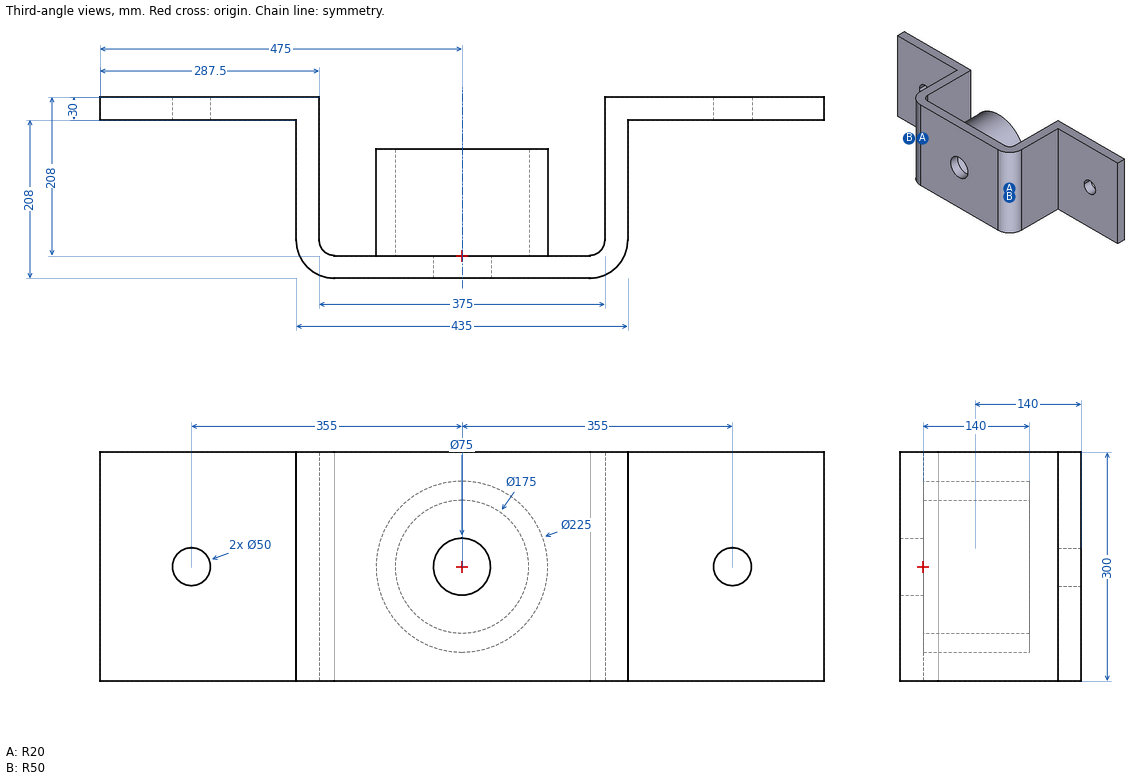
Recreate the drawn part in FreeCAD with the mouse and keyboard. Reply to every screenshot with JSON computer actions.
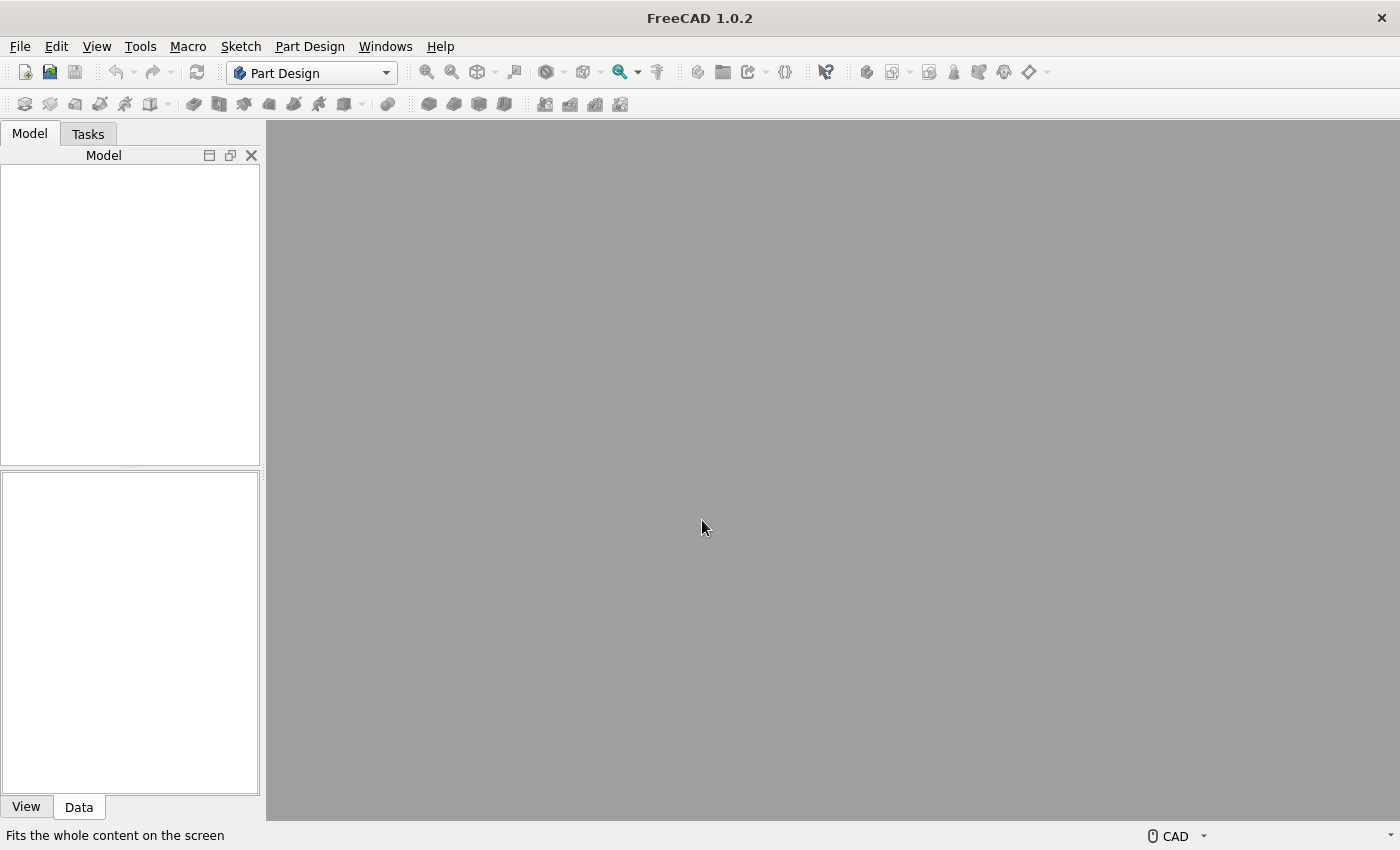
{"action": "left_click", "coordinate": [25, 72]}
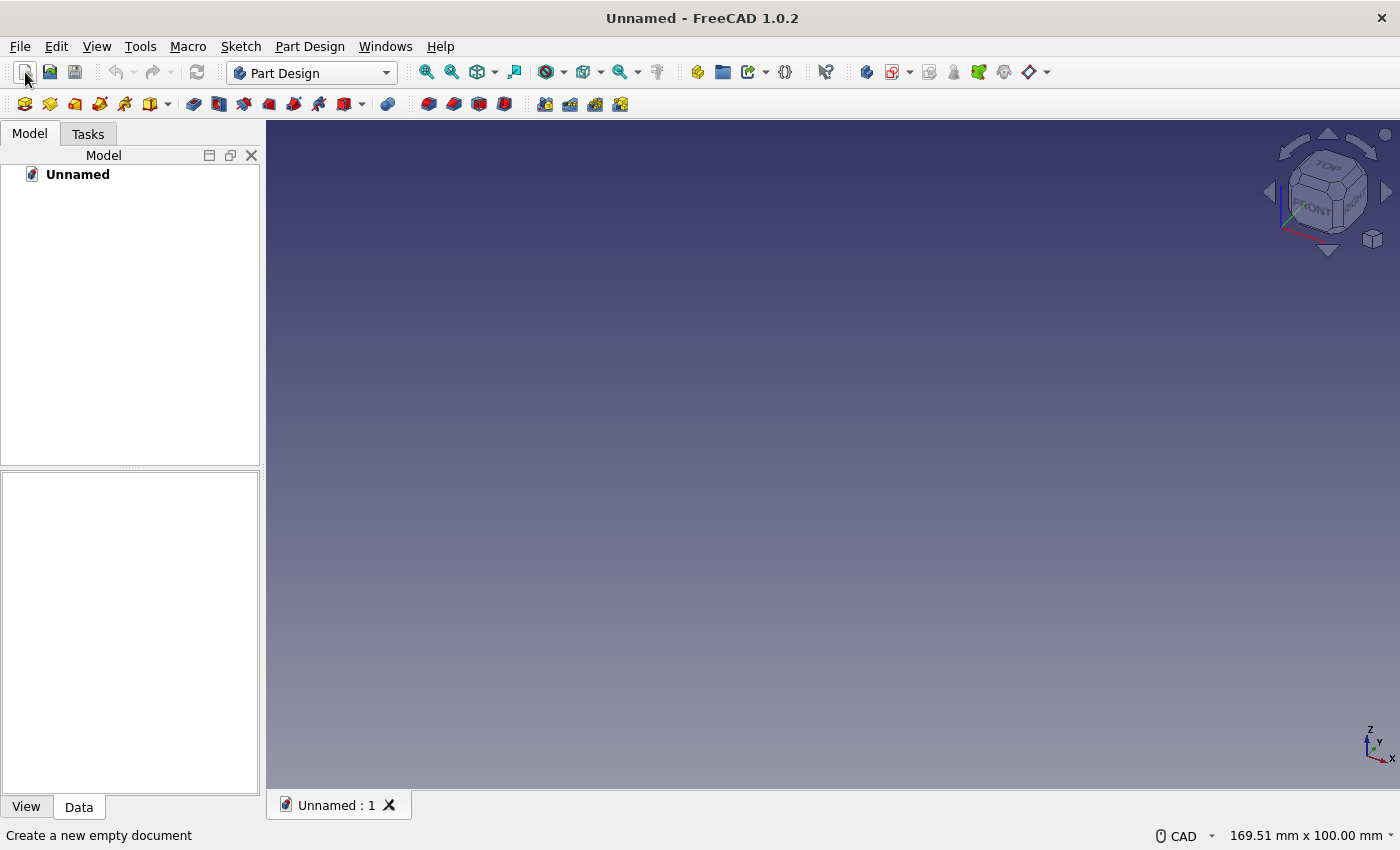
{"action": "left_click", "coordinate": [892, 72]}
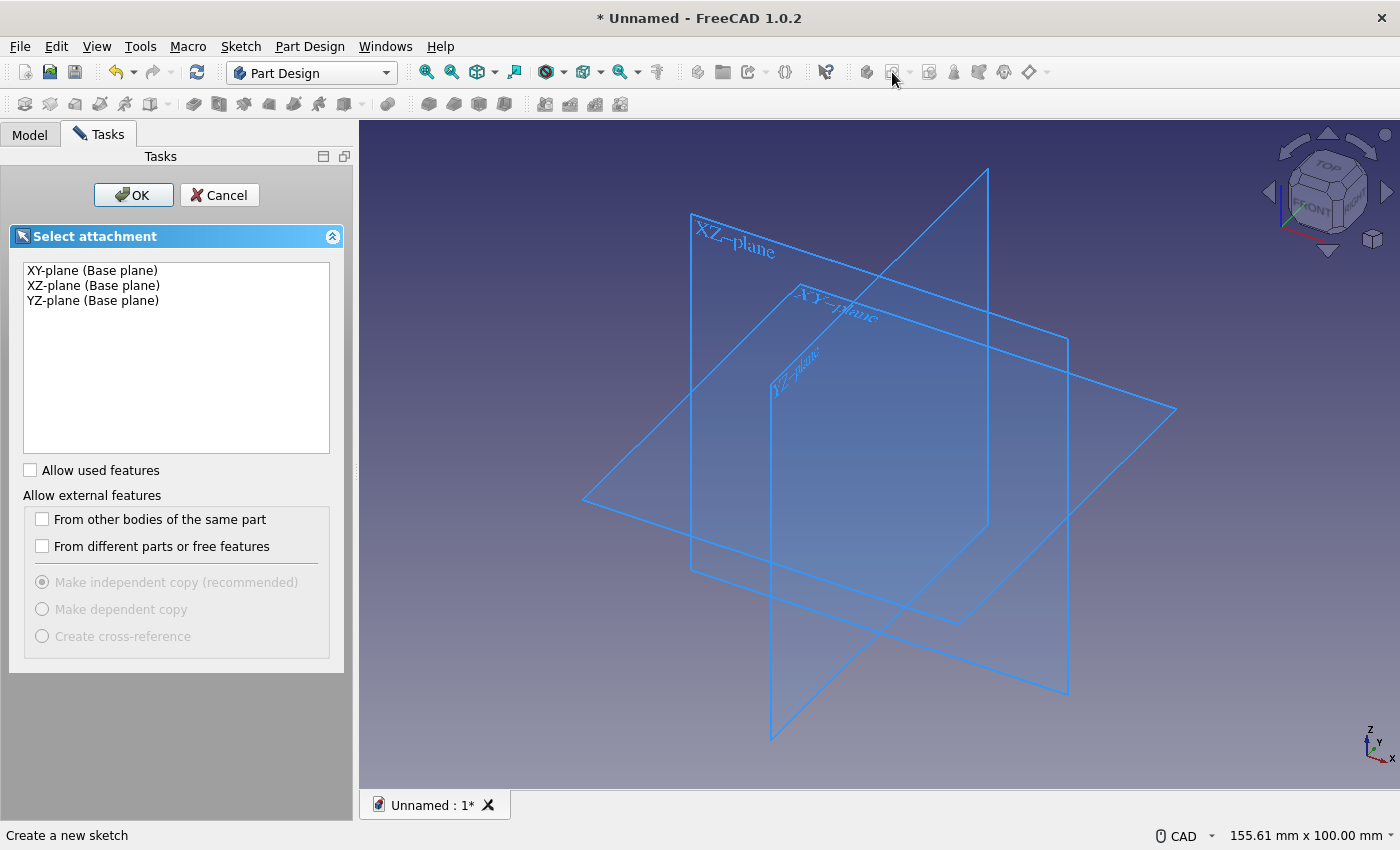
{"action": "left_click", "coordinate": [84, 270]}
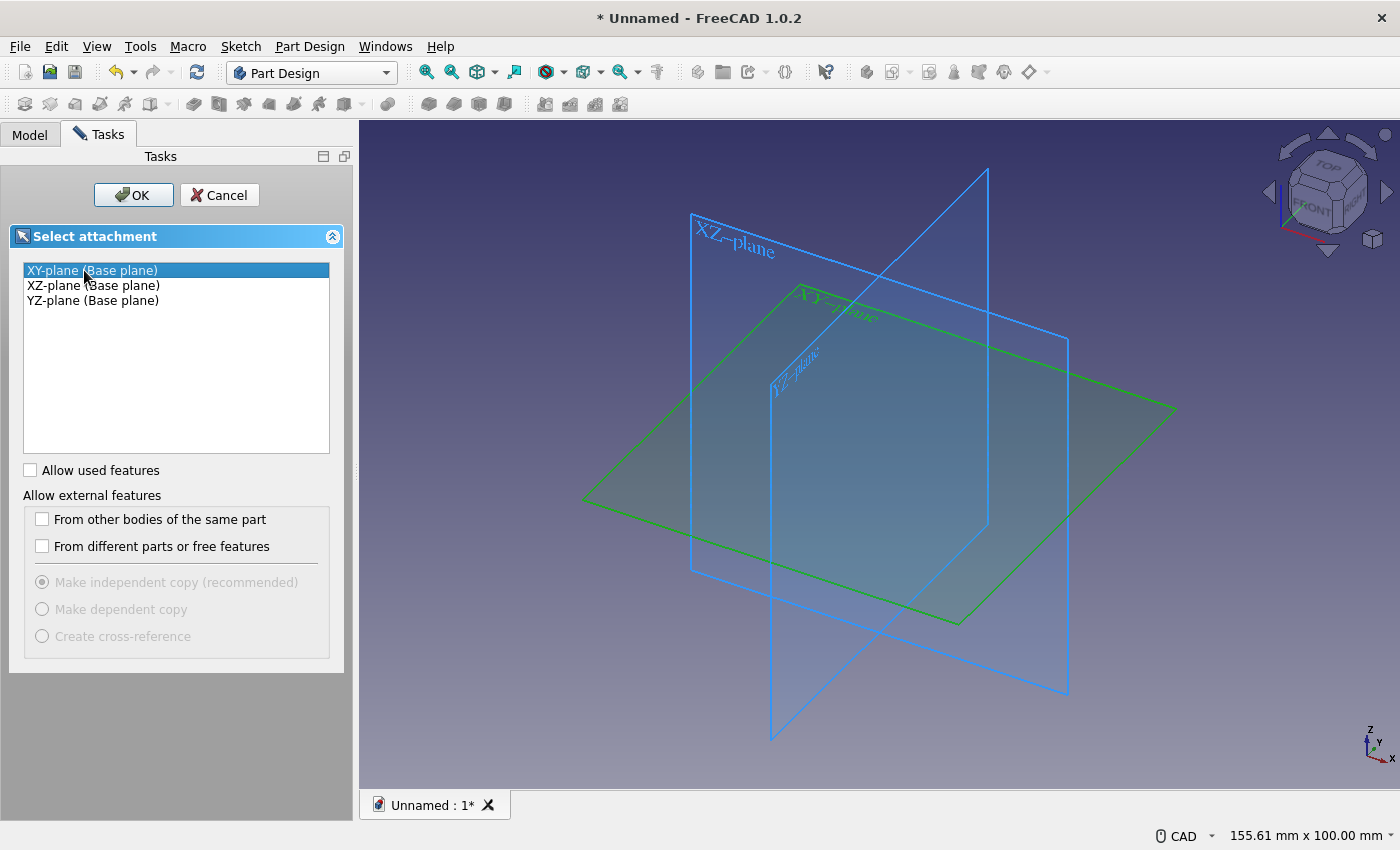
{"action": "left_click", "coordinate": [134, 195]}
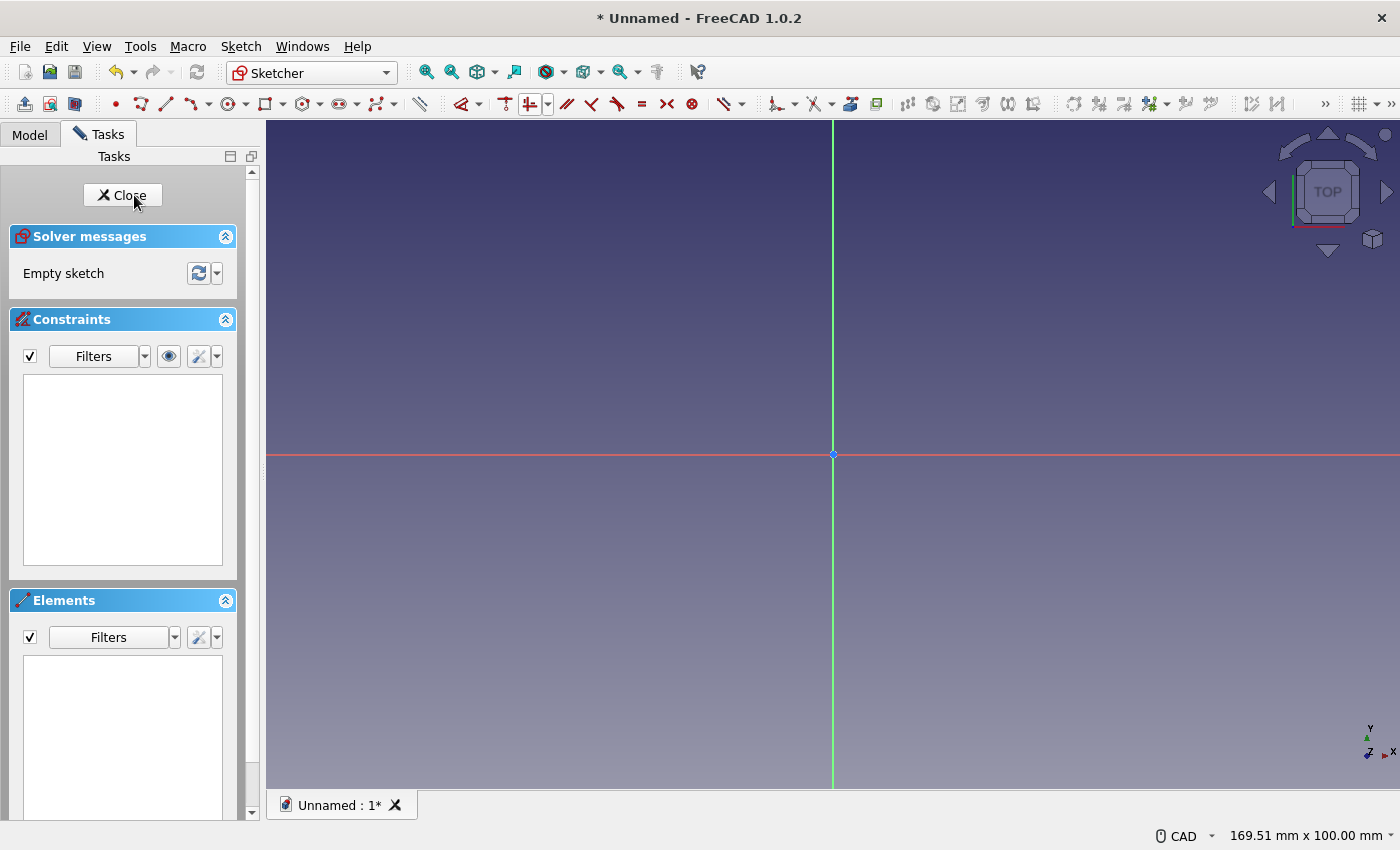
{"action": "scroll", "coordinate": [756, 529], "scroll_direction": "down", "scroll_amount": 11}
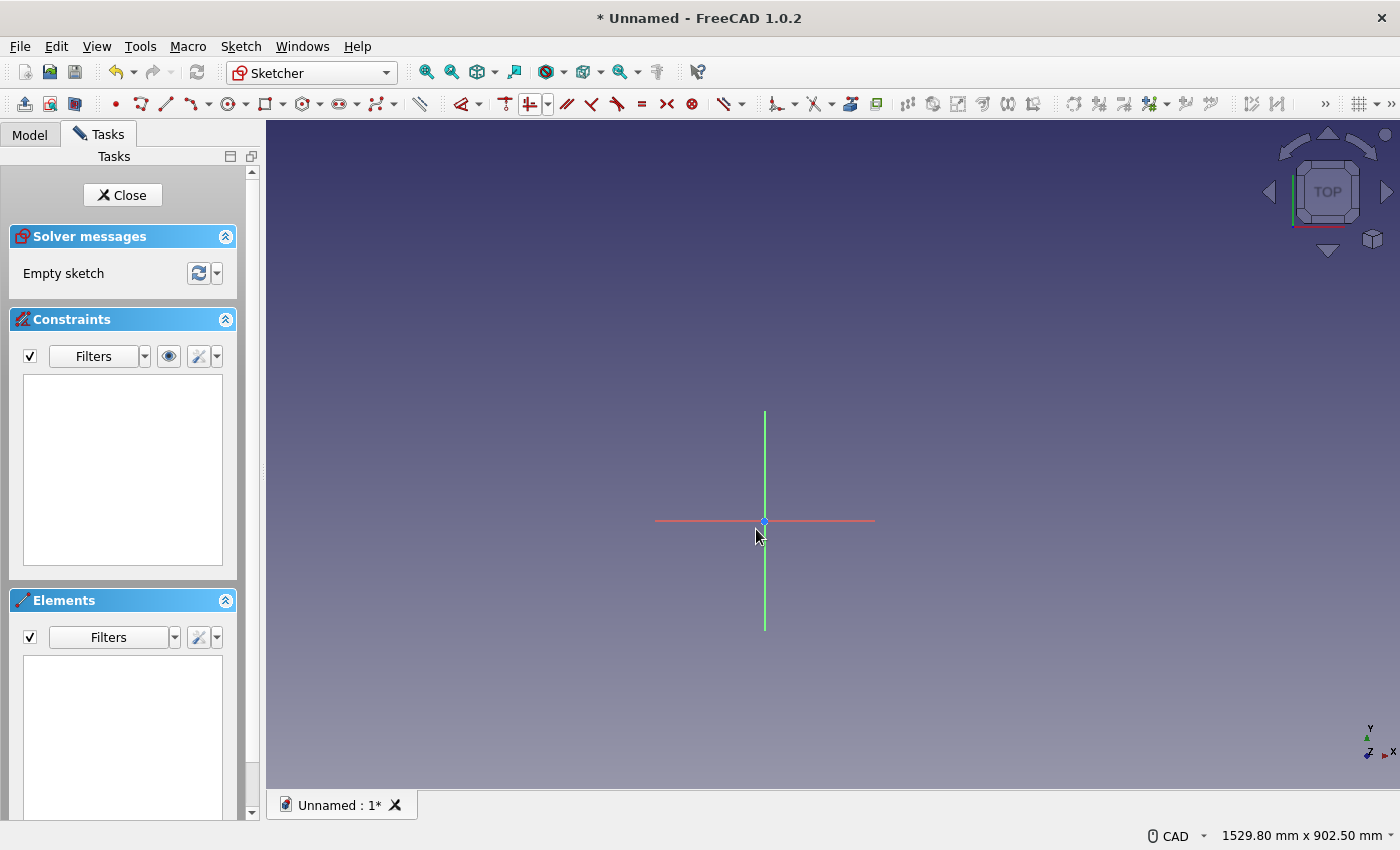
{"action": "left_click", "coordinate": [141, 104]}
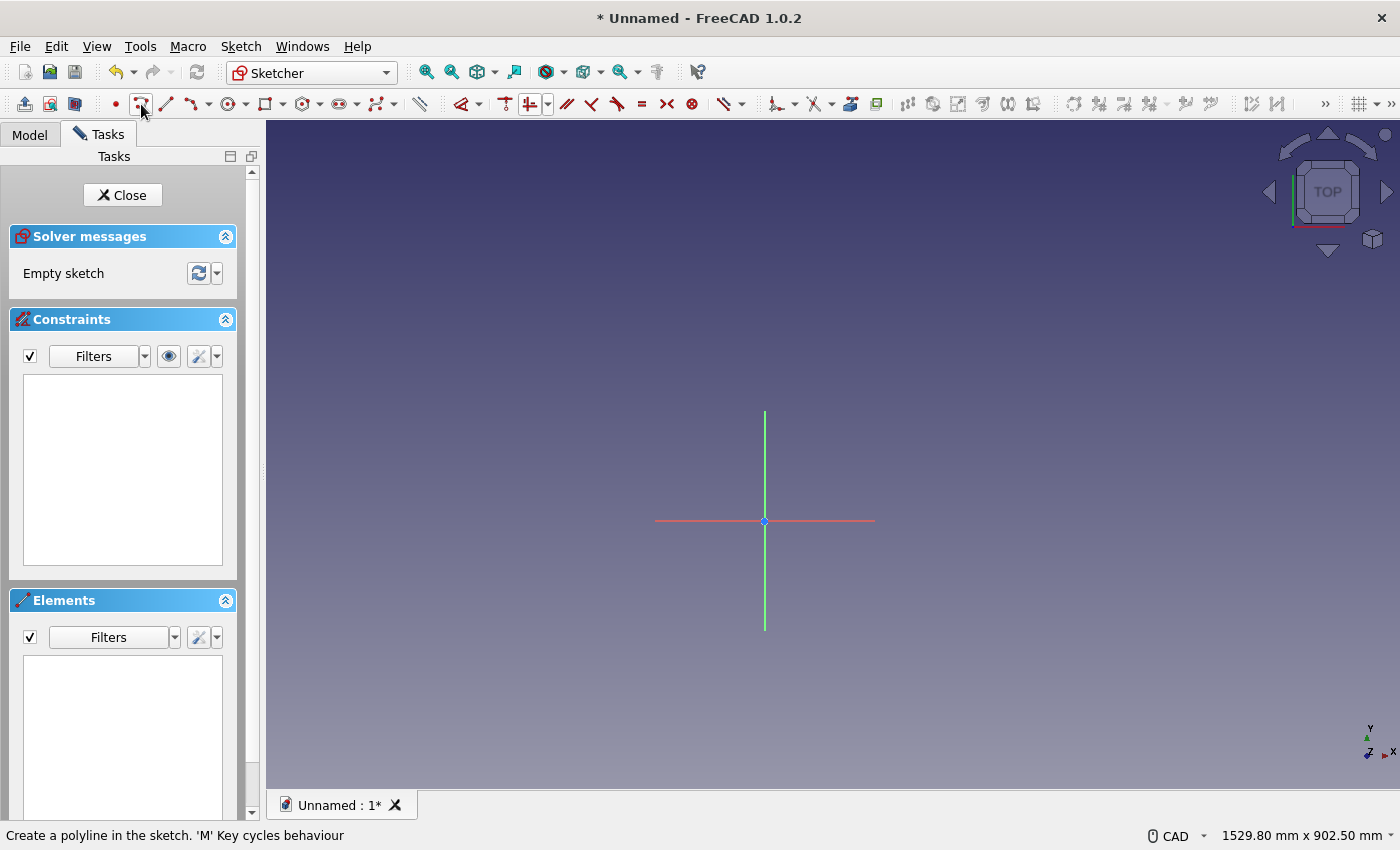
{"action": "left_click", "coordinate": [904, 521]}
{"action": "left_click", "coordinate": [626, 512]}
{"action": "left_click", "coordinate": [626, 367]}
{"action": "left_click", "coordinate": [413, 367]}
{"action": "left_click", "coordinate": [413, 389]}
{"action": "left_click", "coordinate": [604, 389]}
{"action": "left_click", "coordinate": [604, 544]}
{"action": "left_click", "coordinate": [926, 544]}
{"action": "left_click", "coordinate": [926, 389]}
{"action": "left_click", "coordinate": [1117, 389]}
{"action": "left_click", "coordinate": [1117, 367]}
{"action": "left_click", "coordinate": [904, 367]}
{"action": "left_click", "coordinate": [904, 522]}
{"action": "key", "text": "Escape"}
{"action": "key", "text": "Escape"}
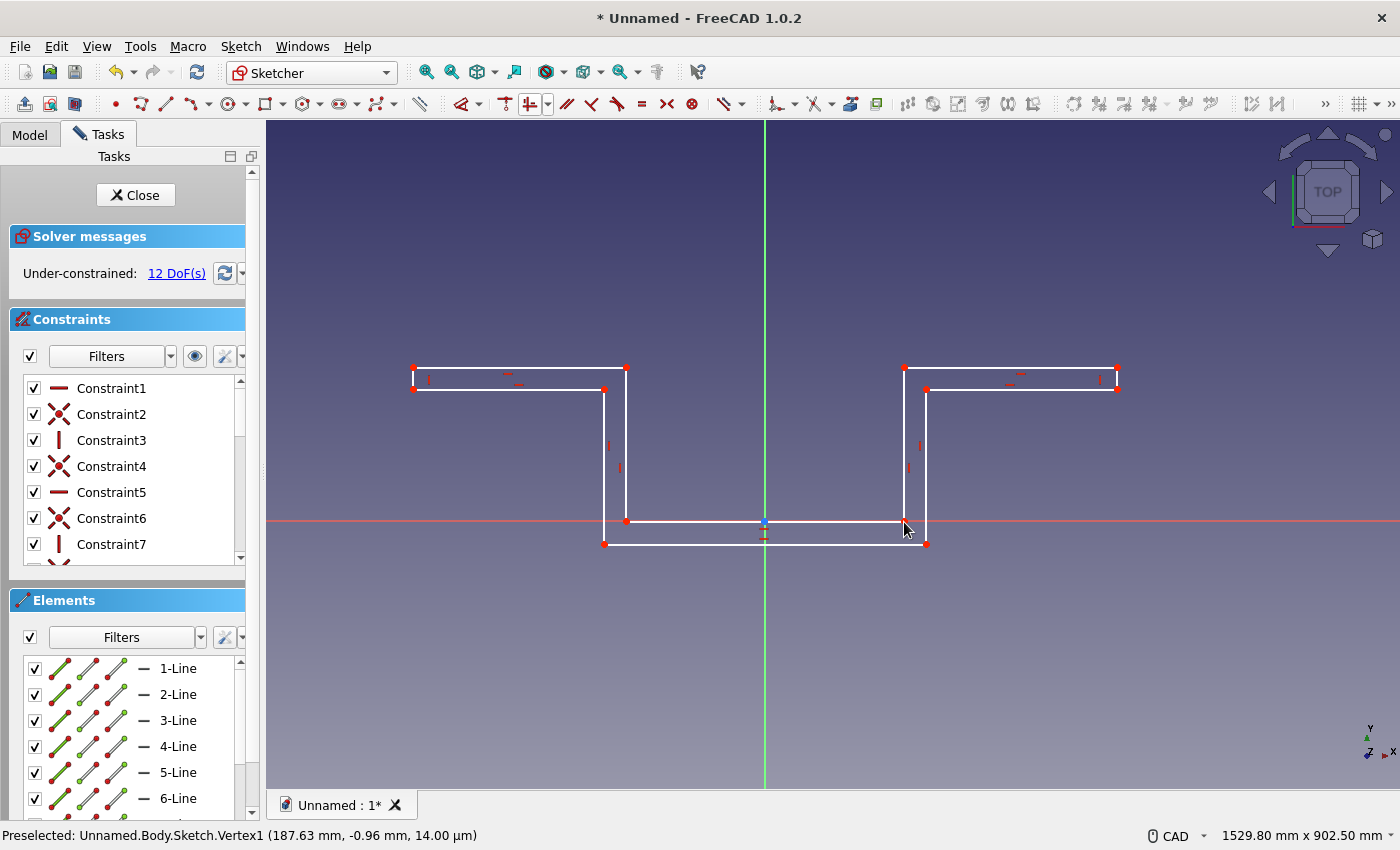
{"action": "left_click", "coordinate": [604, 390]}